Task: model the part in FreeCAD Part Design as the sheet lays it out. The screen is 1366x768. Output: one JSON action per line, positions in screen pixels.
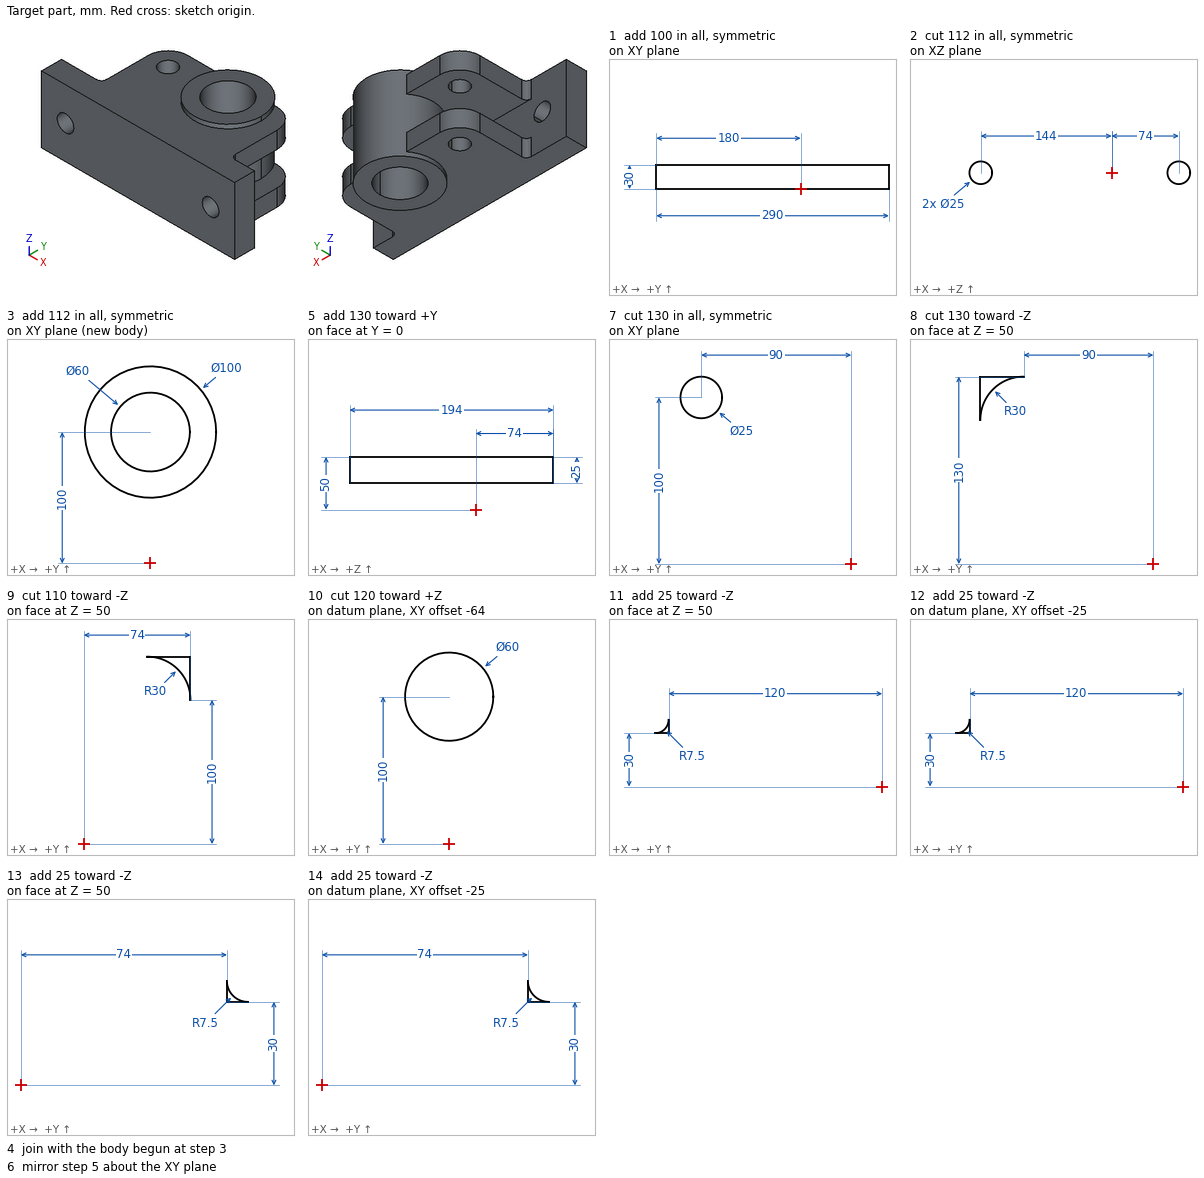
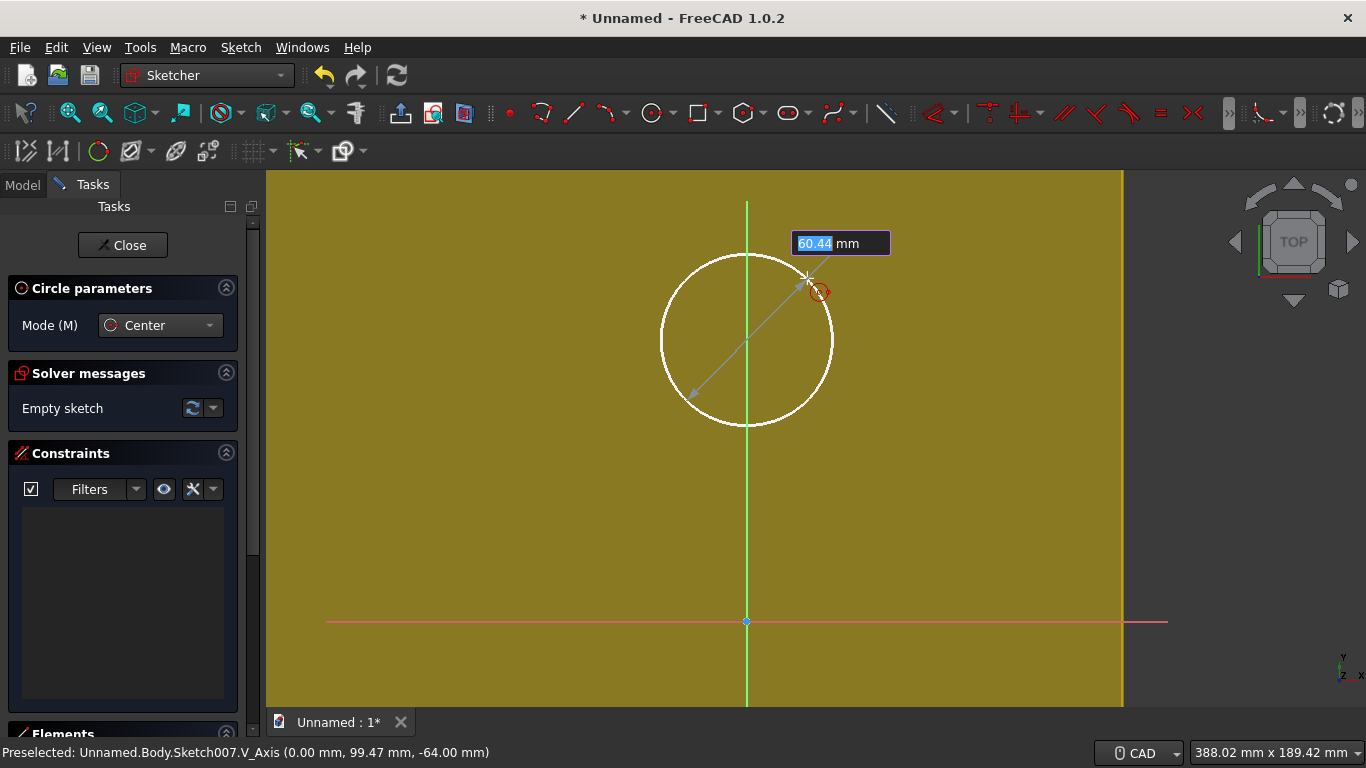
{"action": "type", "text": "60"}
{"action": "key", "text": "Return"}
{"action": "key", "text": "Escape"}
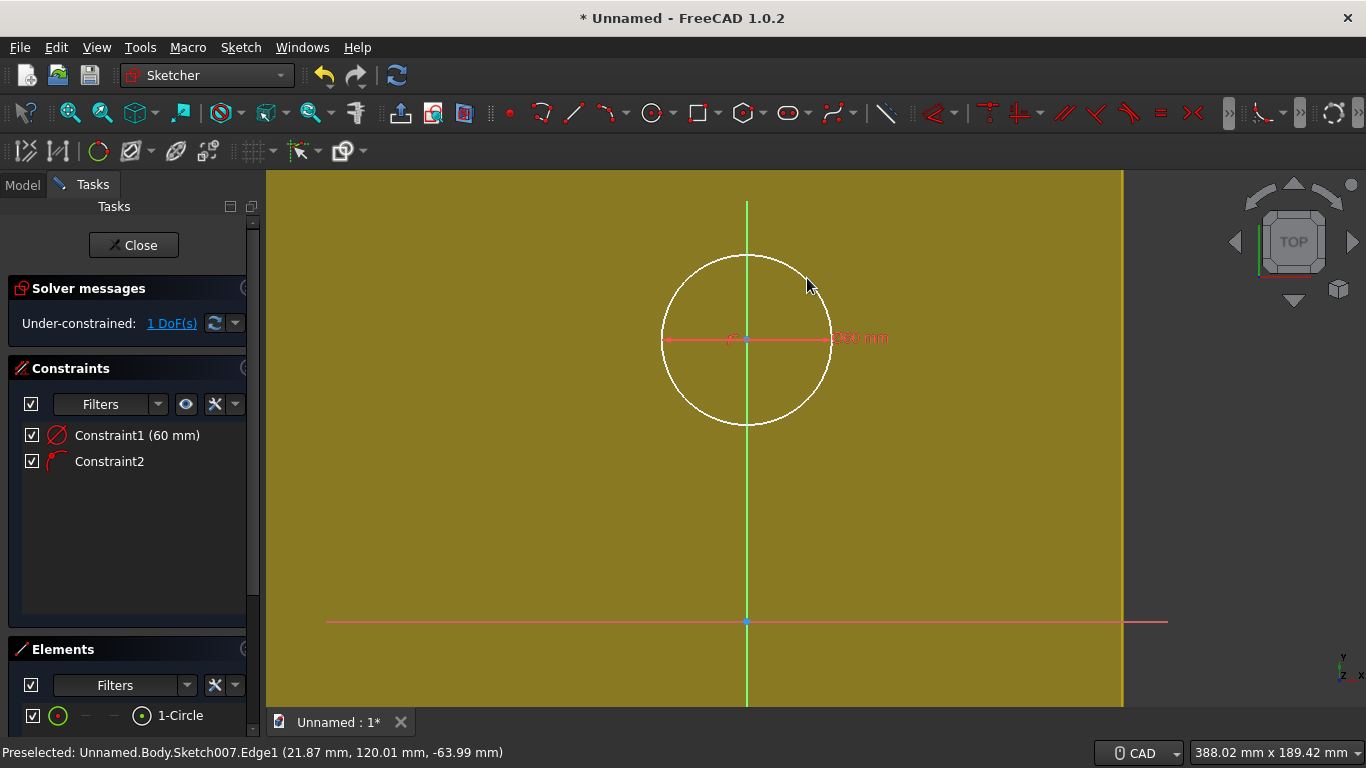
{"action": "left_click", "coordinate": [934, 114]}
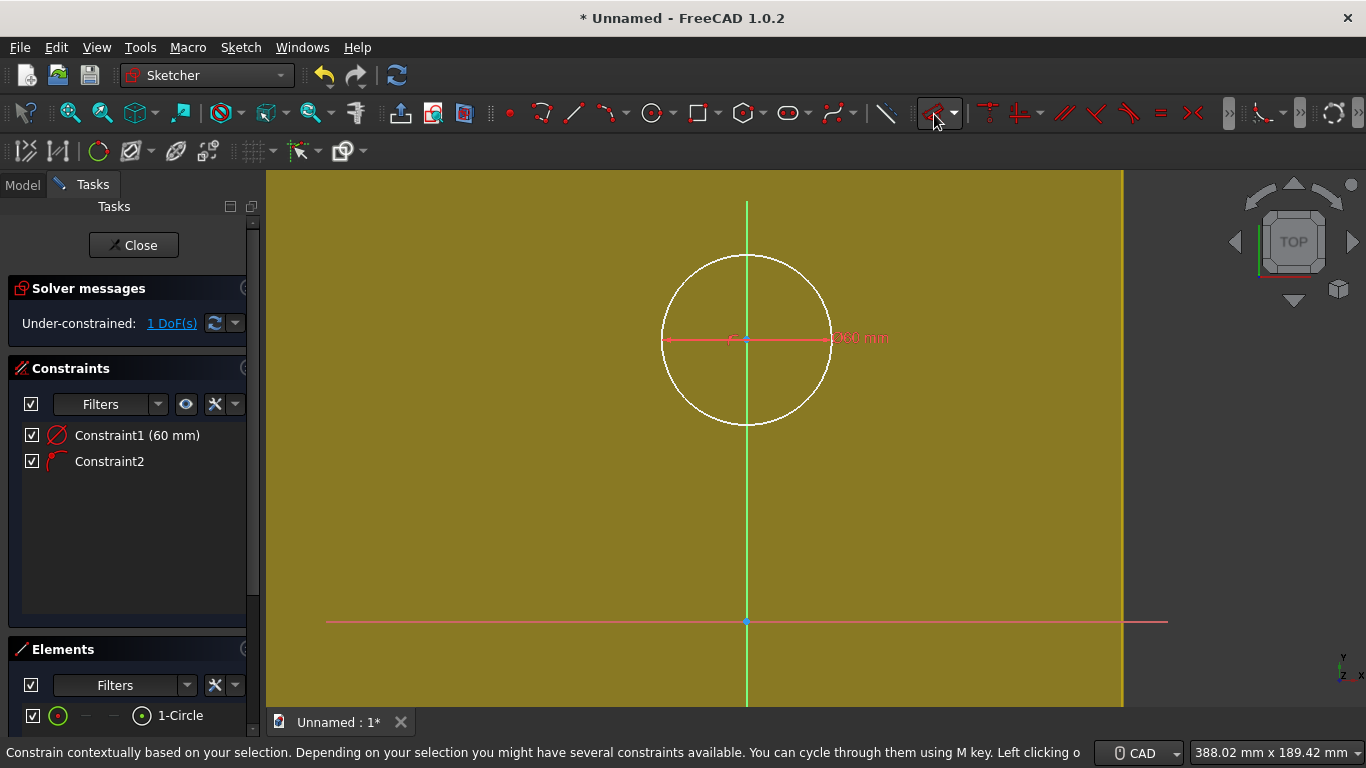
{"action": "left_click", "coordinate": [747, 340]}
{"action": "left_click", "coordinate": [781, 481]}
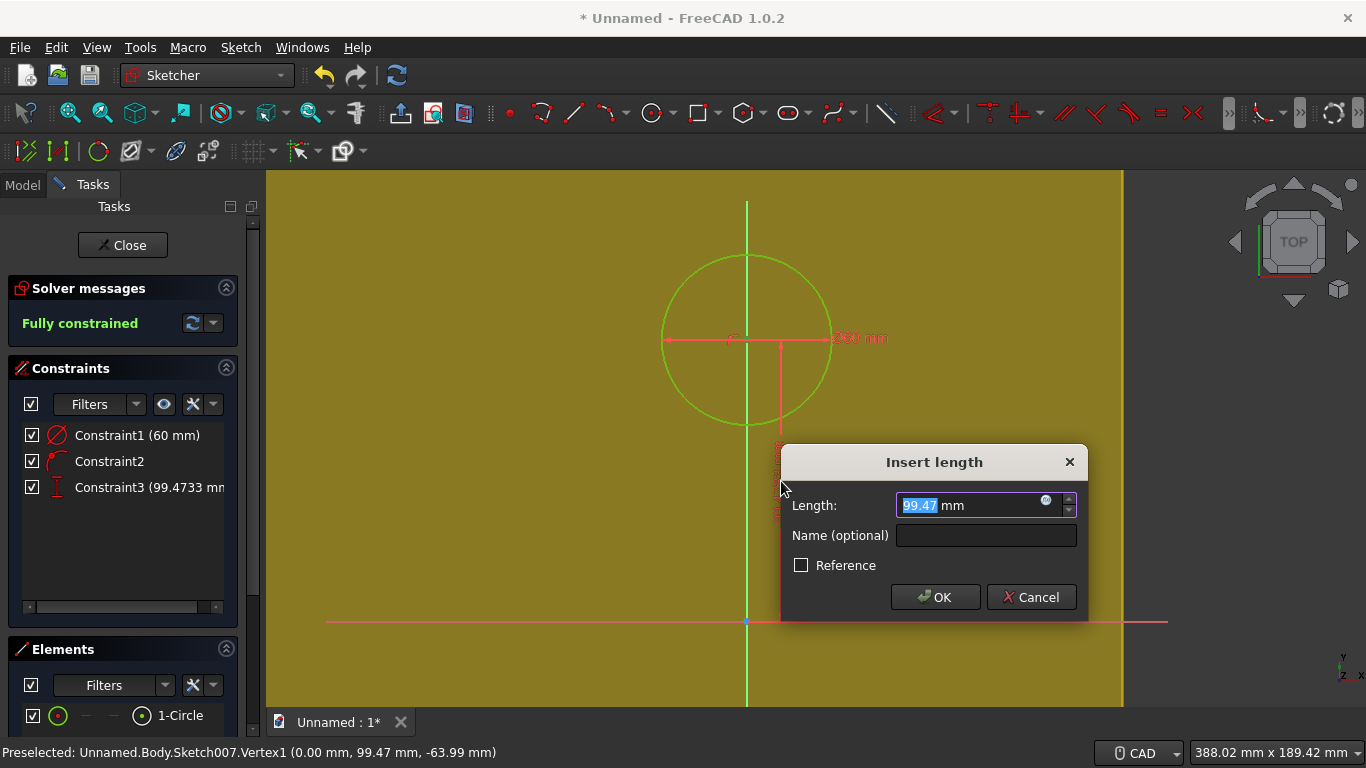
{"action": "type", "text": "100"}
{"action": "key", "text": "Return"}
{"action": "key", "text": "Escape"}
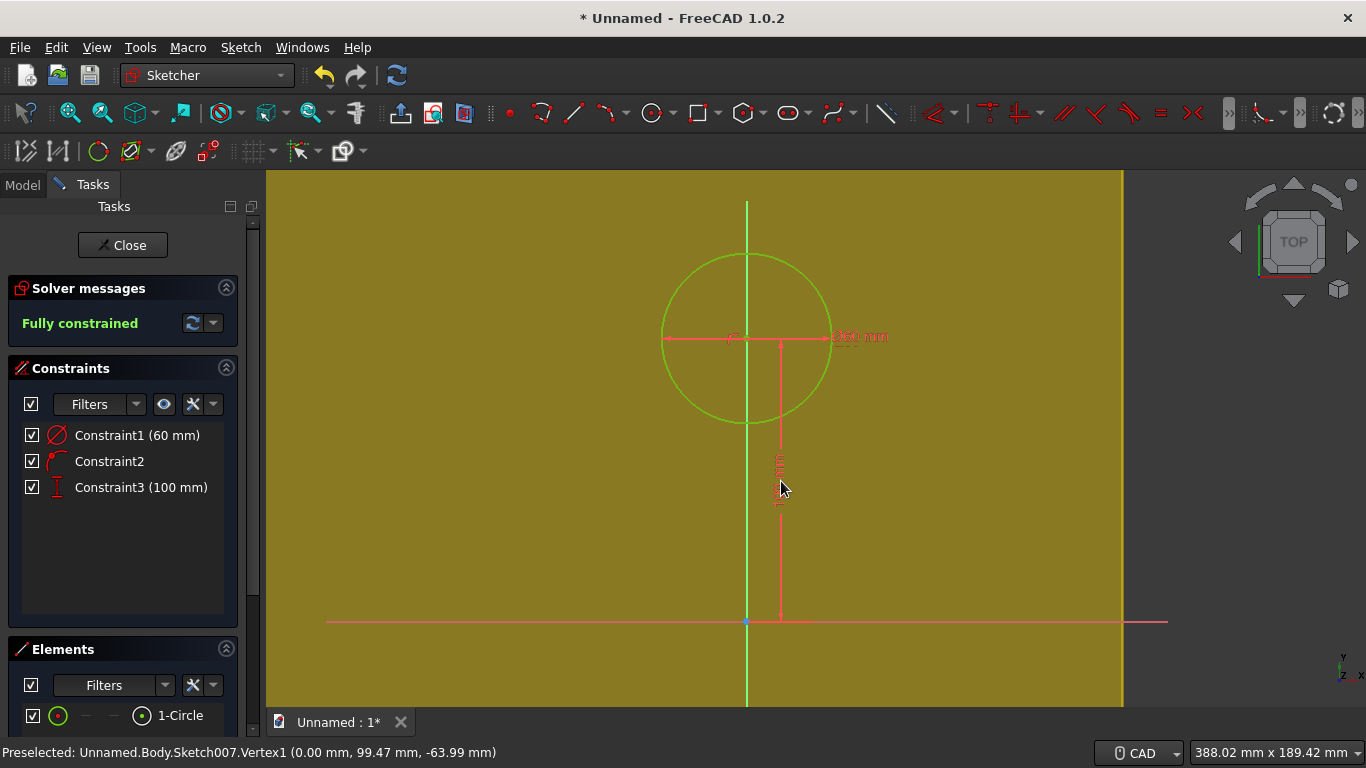
{"action": "left_click", "coordinate": [123, 245]}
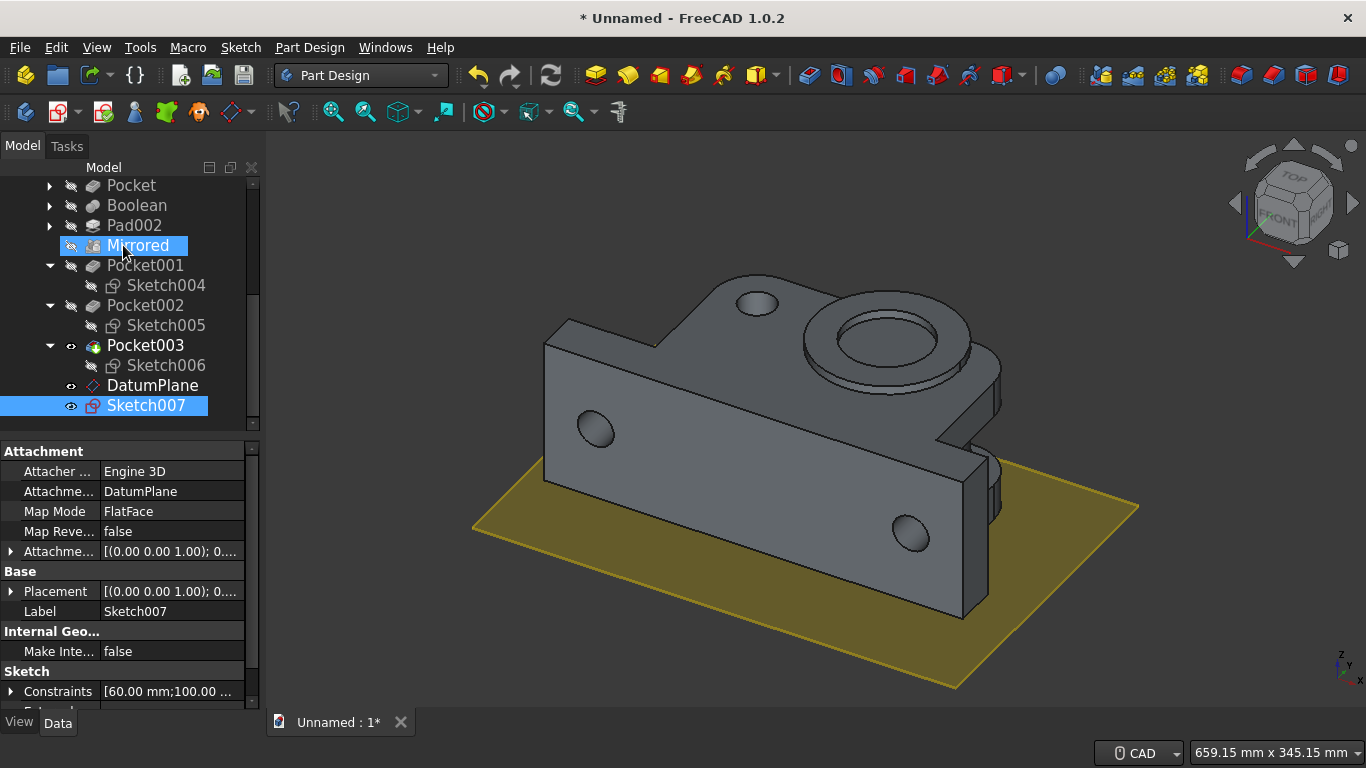
{"action": "left_click", "coordinate": [810, 76]}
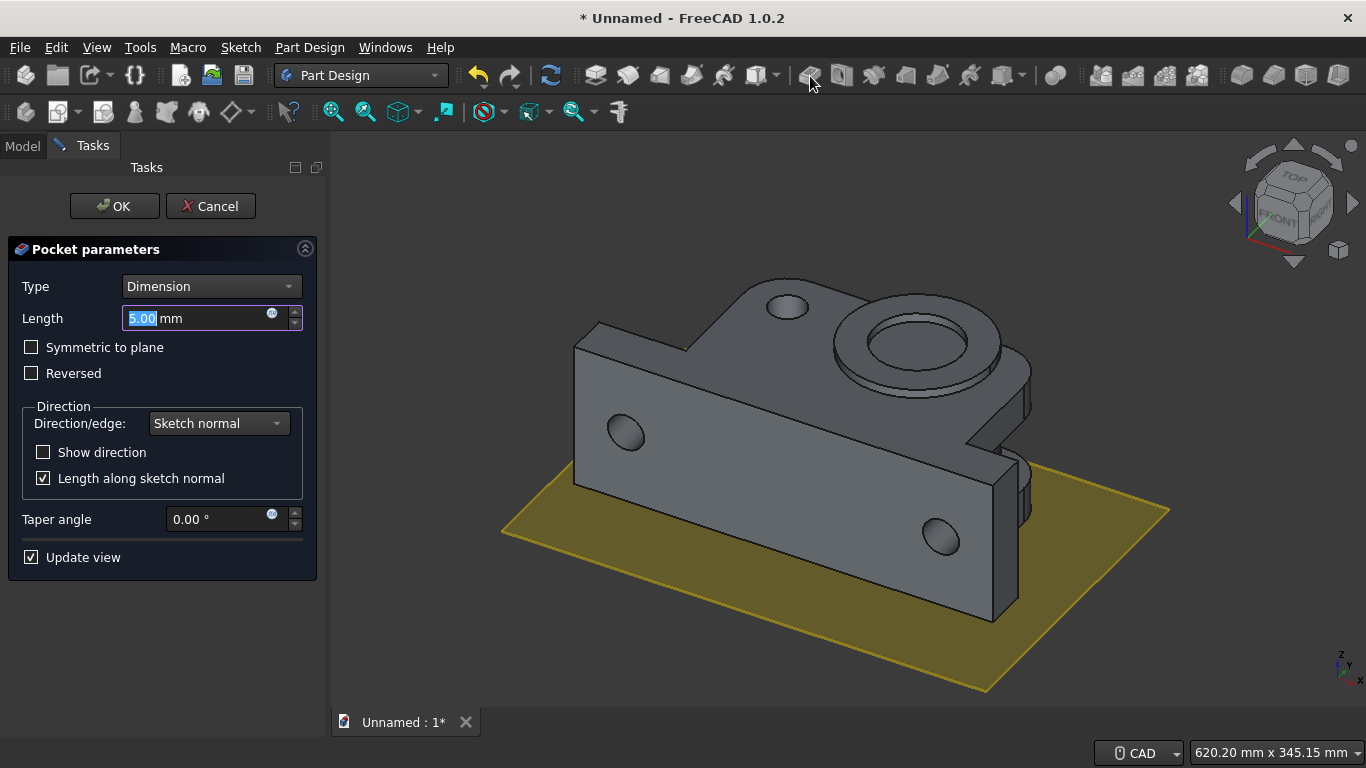
{"action": "type", "text": "120"}
{"action": "key", "text": "Tab"}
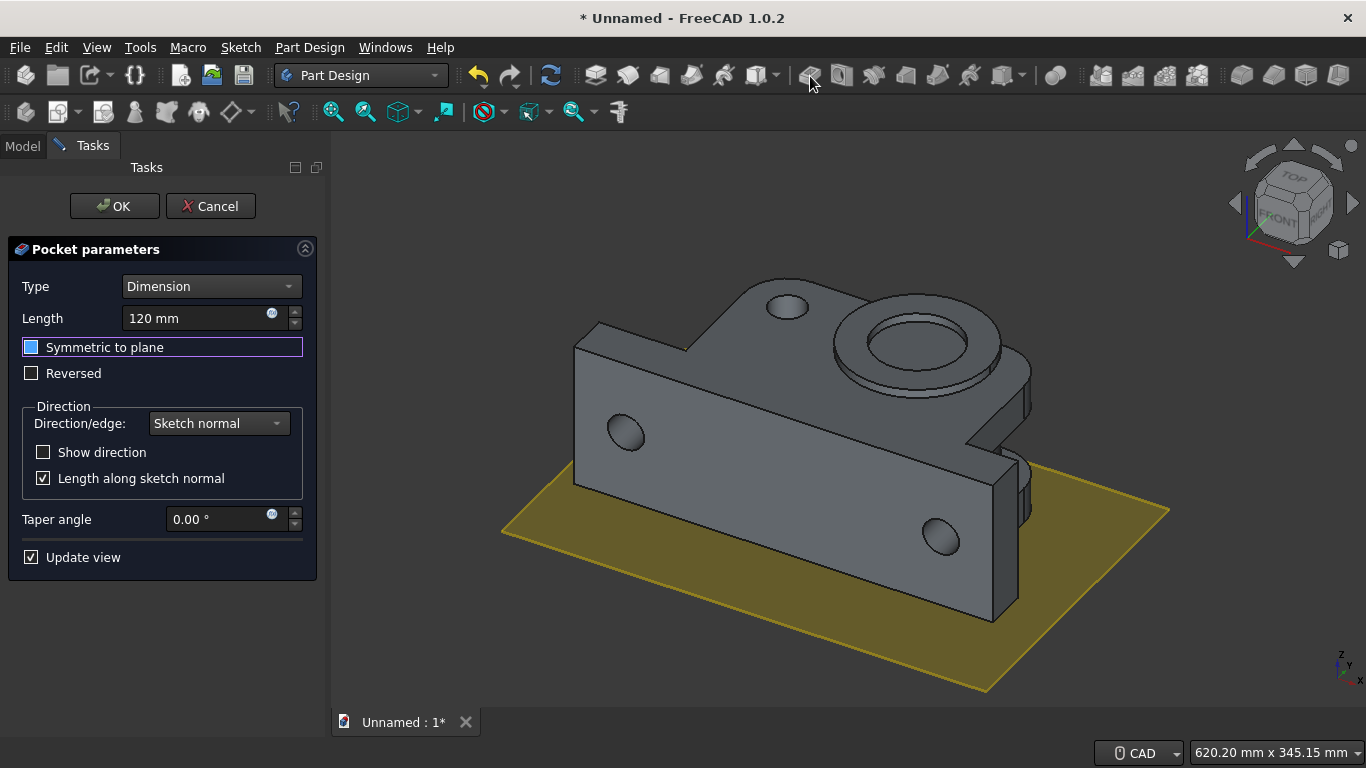
{"action": "left_click", "coordinate": [30, 373]}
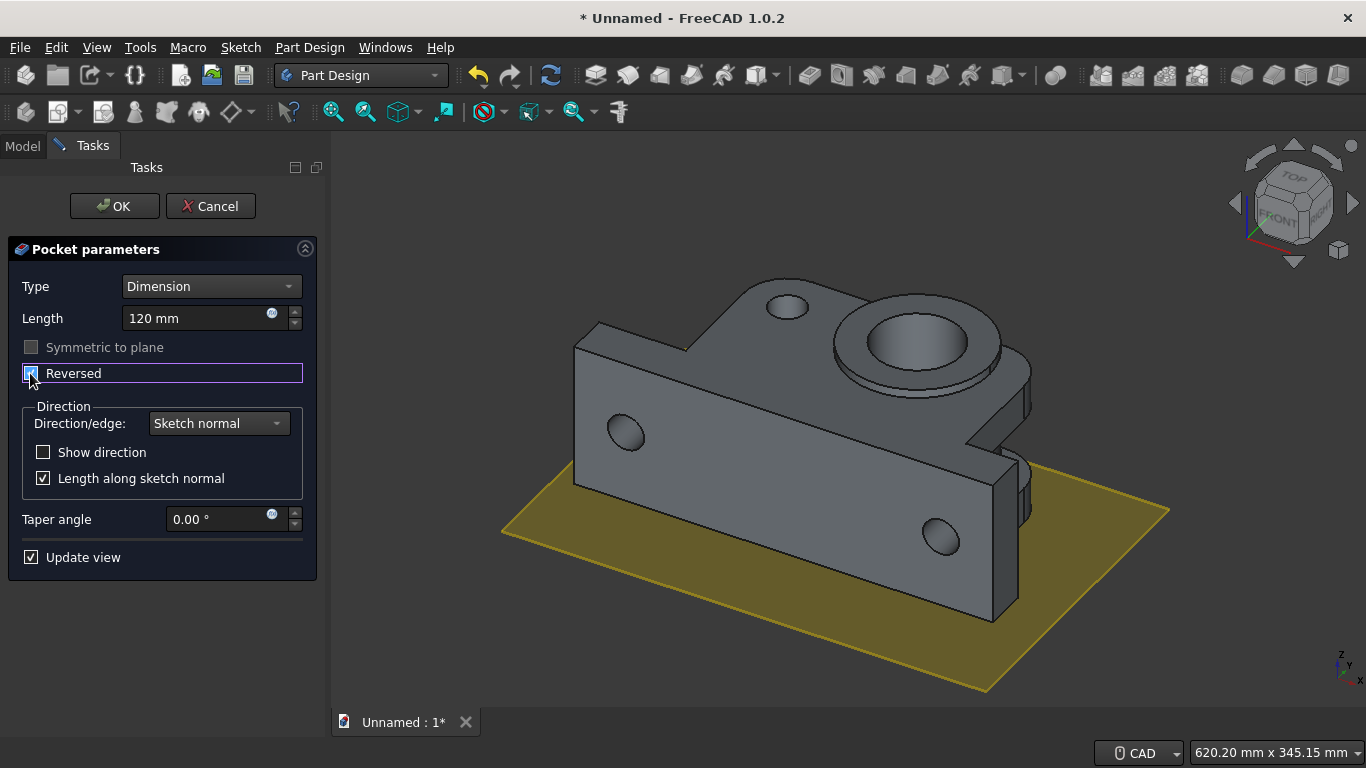
{"action": "left_click", "coordinate": [115, 206]}